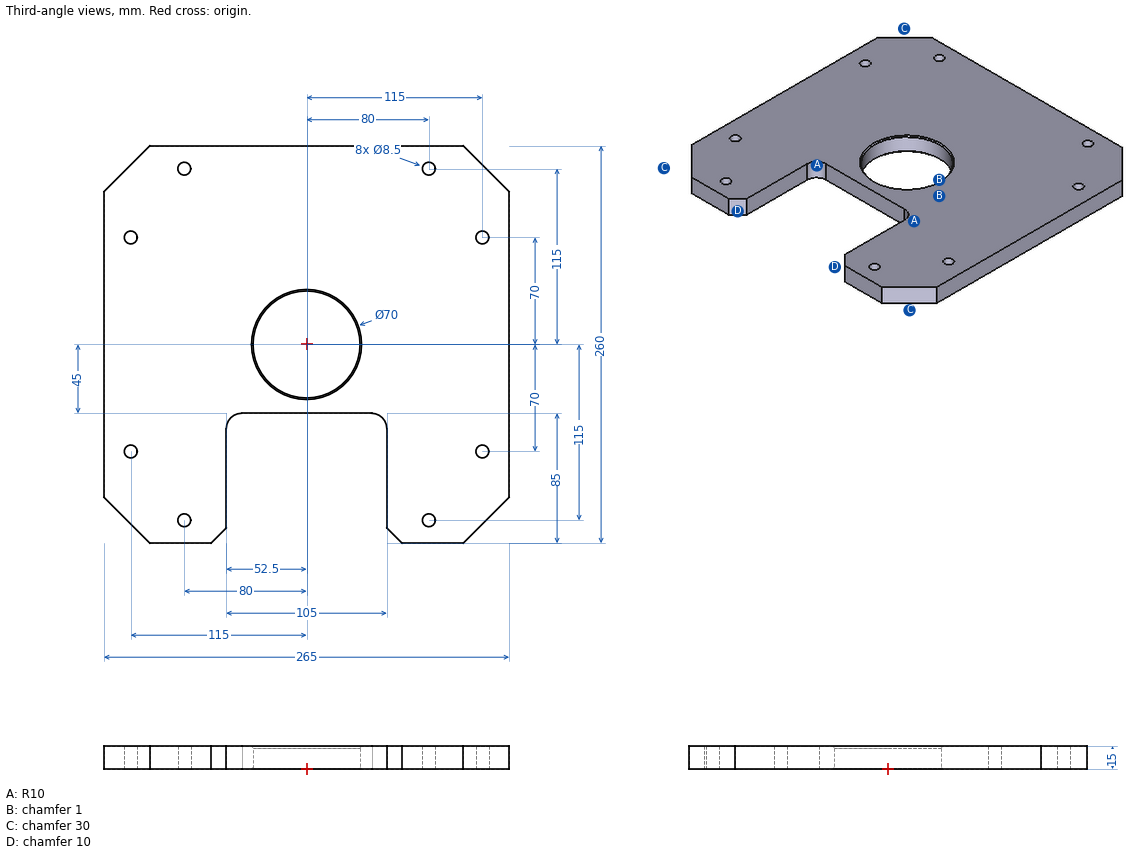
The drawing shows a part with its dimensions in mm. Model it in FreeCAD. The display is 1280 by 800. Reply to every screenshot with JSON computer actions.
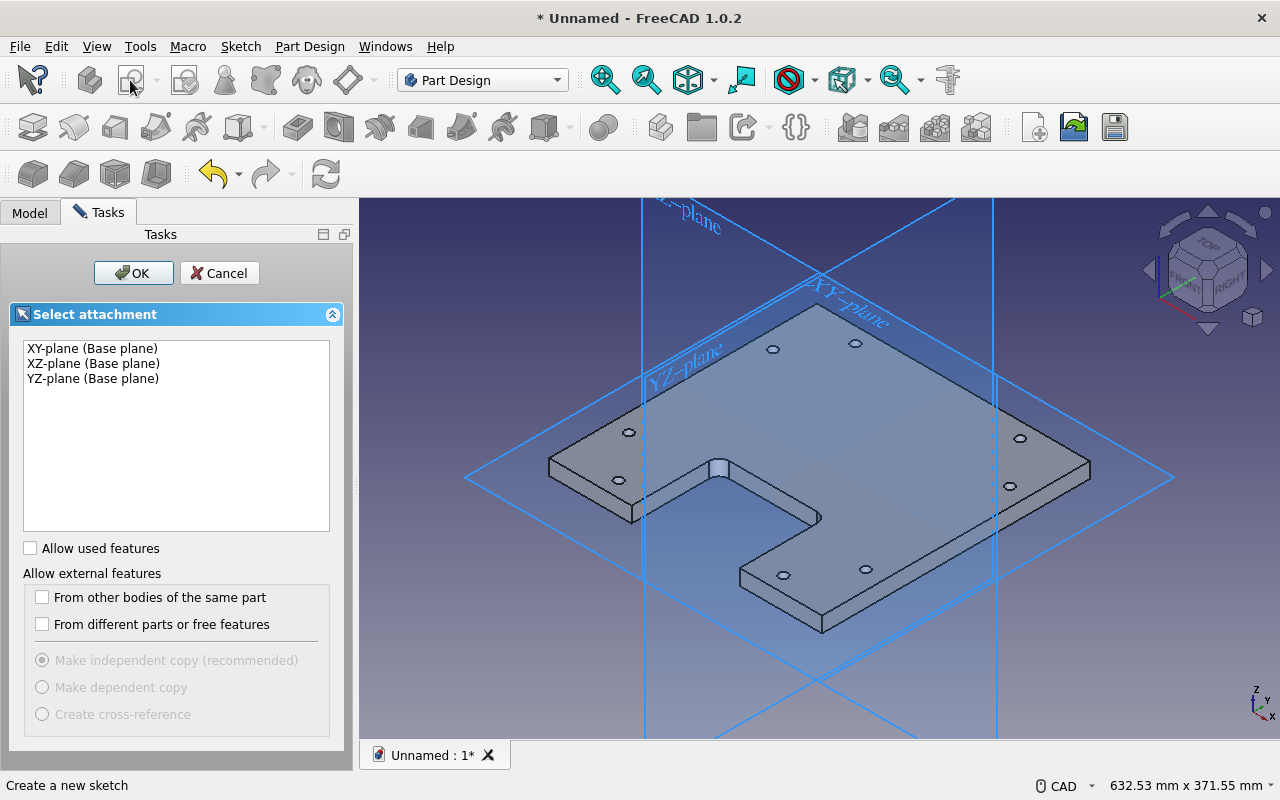
{"action": "left_click", "coordinate": [84, 348]}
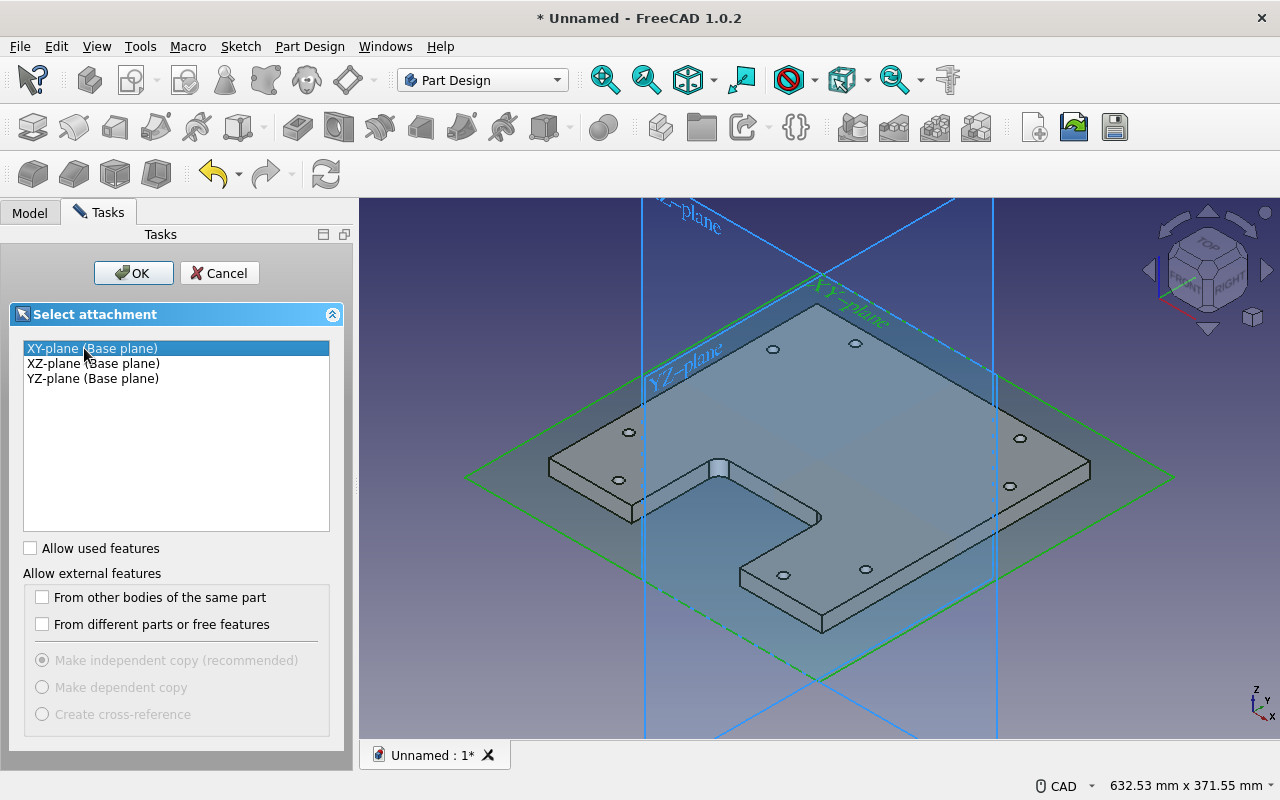
{"action": "left_click", "coordinate": [134, 273]}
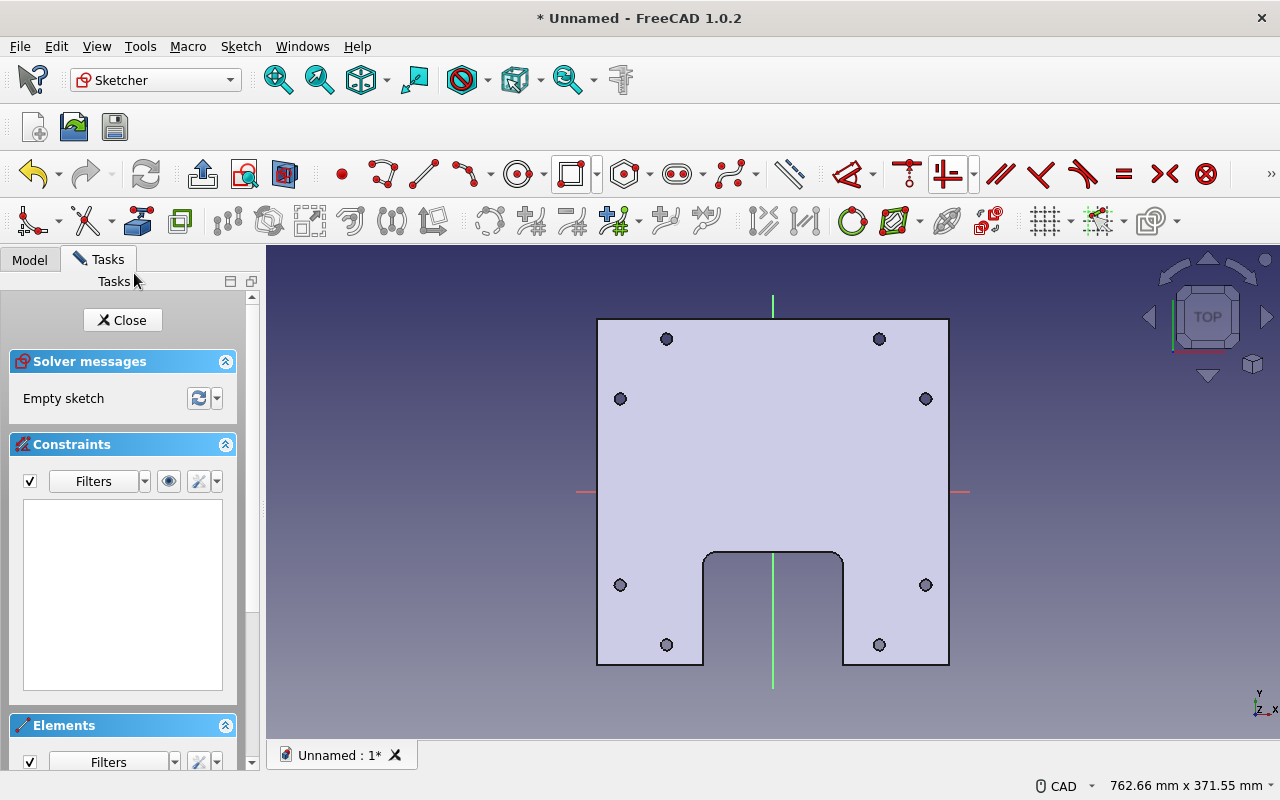
{"action": "key", "text": "q s"}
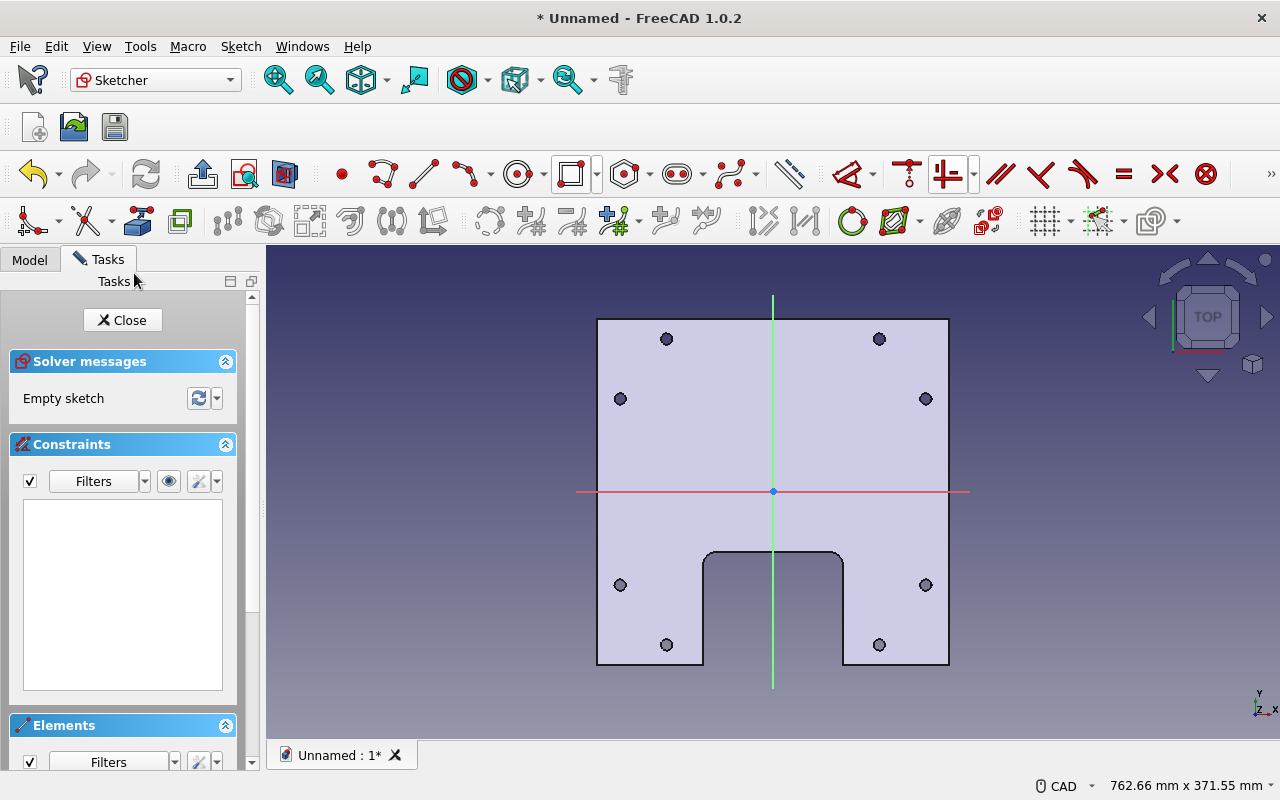
{"action": "scroll", "coordinate": [803, 492], "scroll_direction": "up", "scroll_amount": 6}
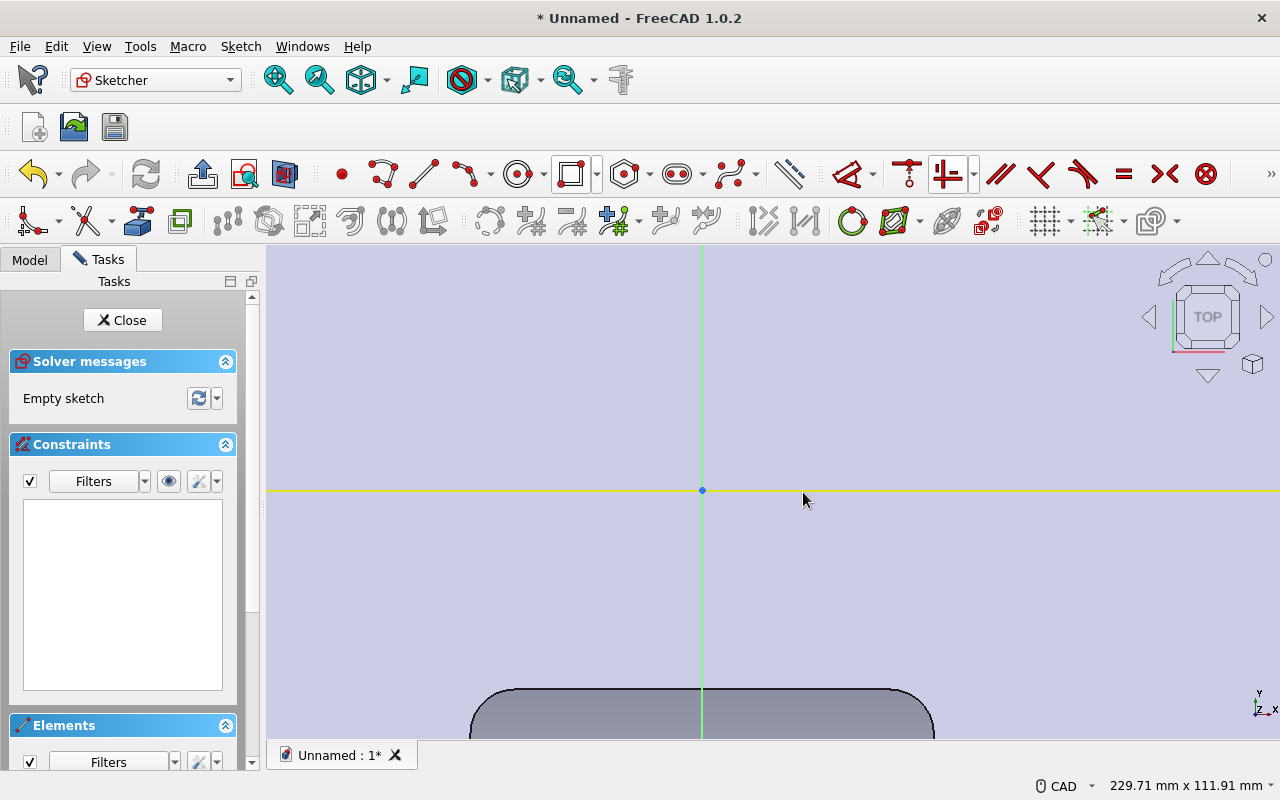
{"action": "left_click", "coordinate": [518, 174]}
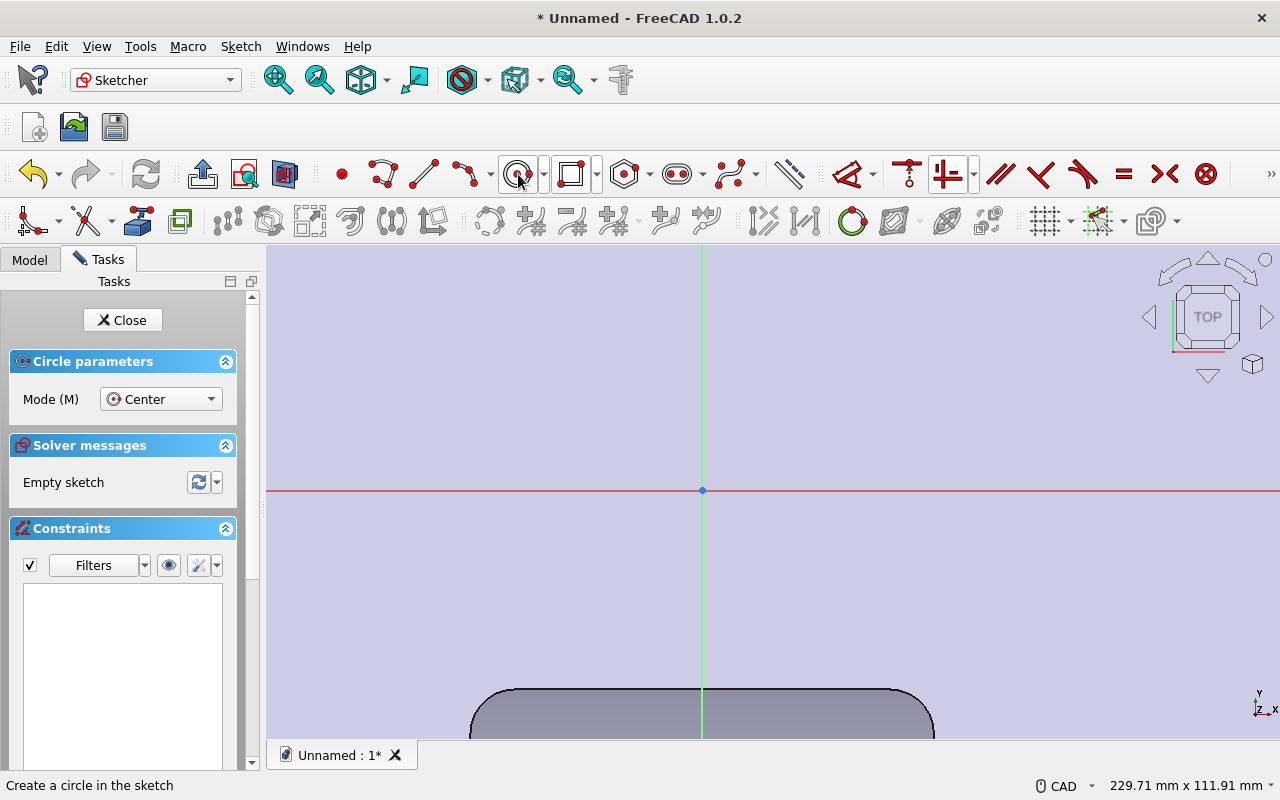
{"action": "left_click", "coordinate": [702, 491]}
{"action": "mouse_move", "coordinate": [811, 382]}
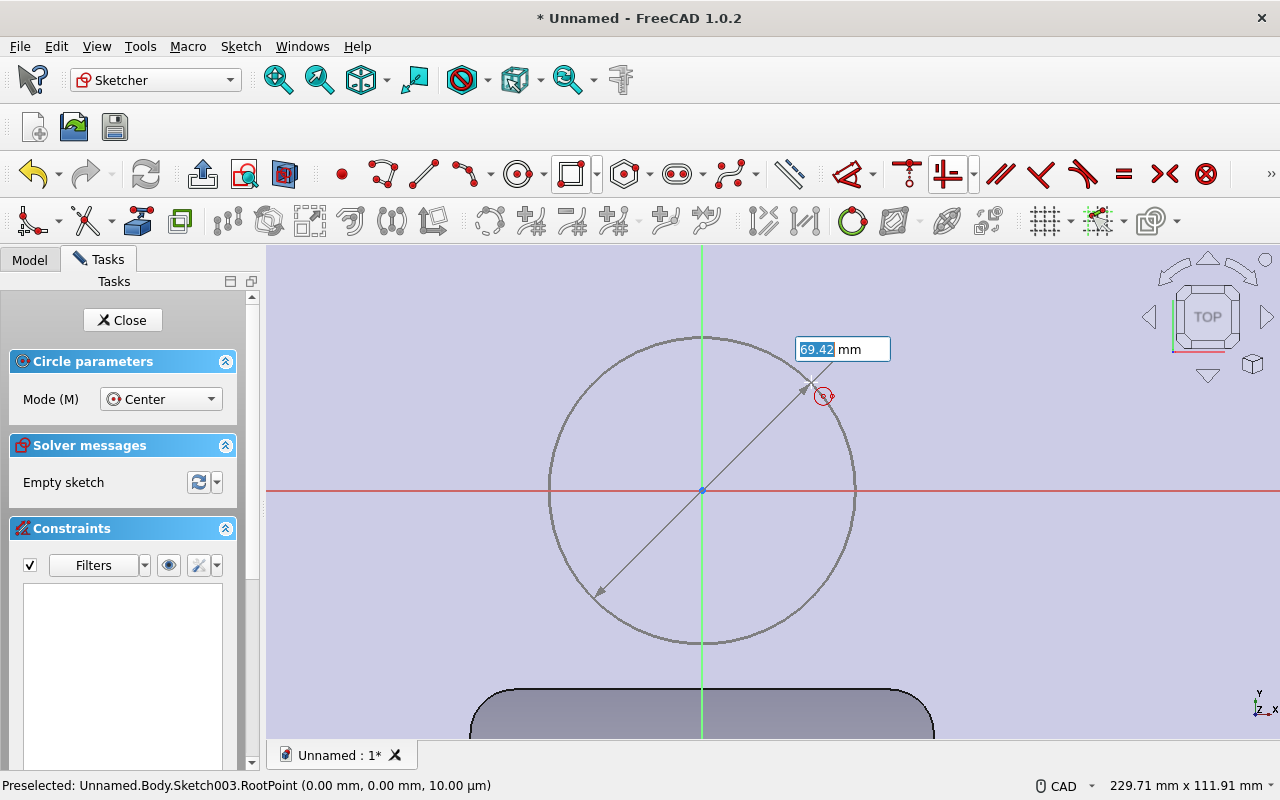
{"action": "type", "text": "70"}
{"action": "key", "text": "Return"}
{"action": "key", "text": "Escape"}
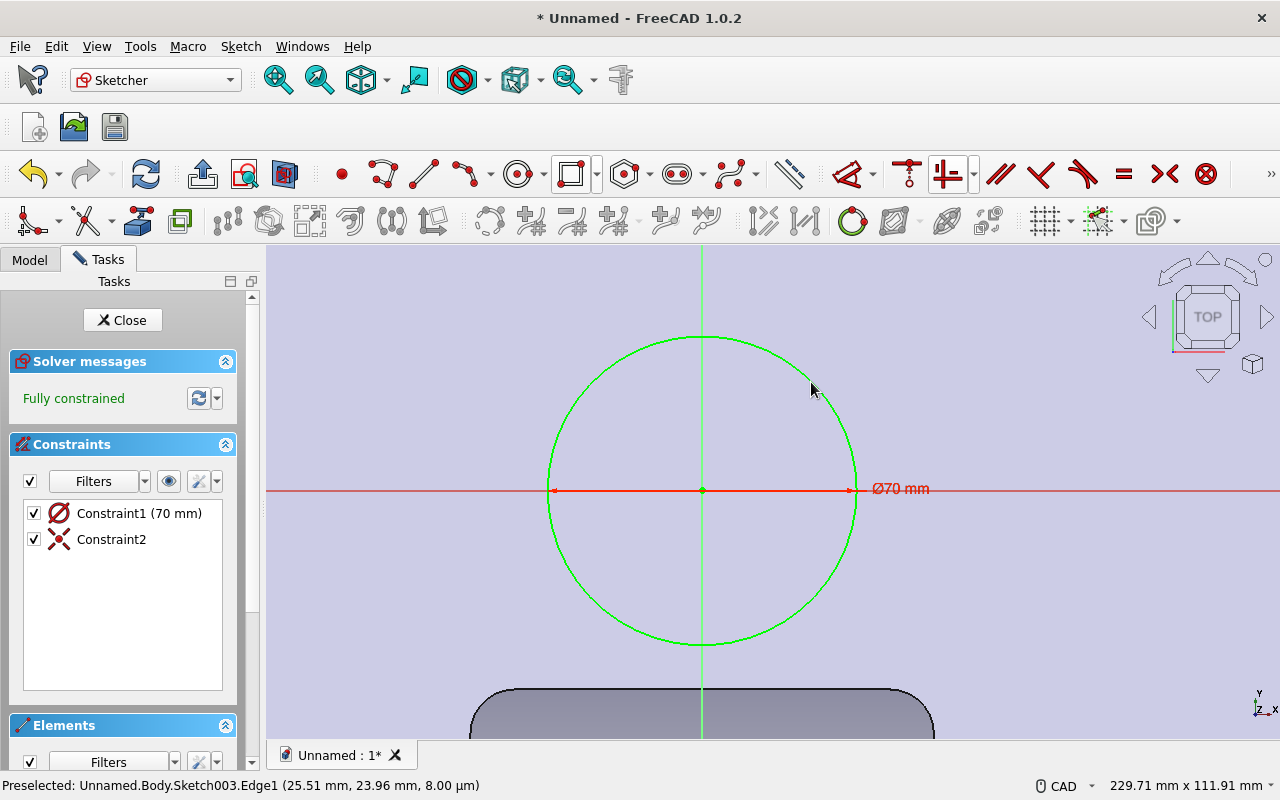
{"action": "left_click", "coordinate": [123, 320]}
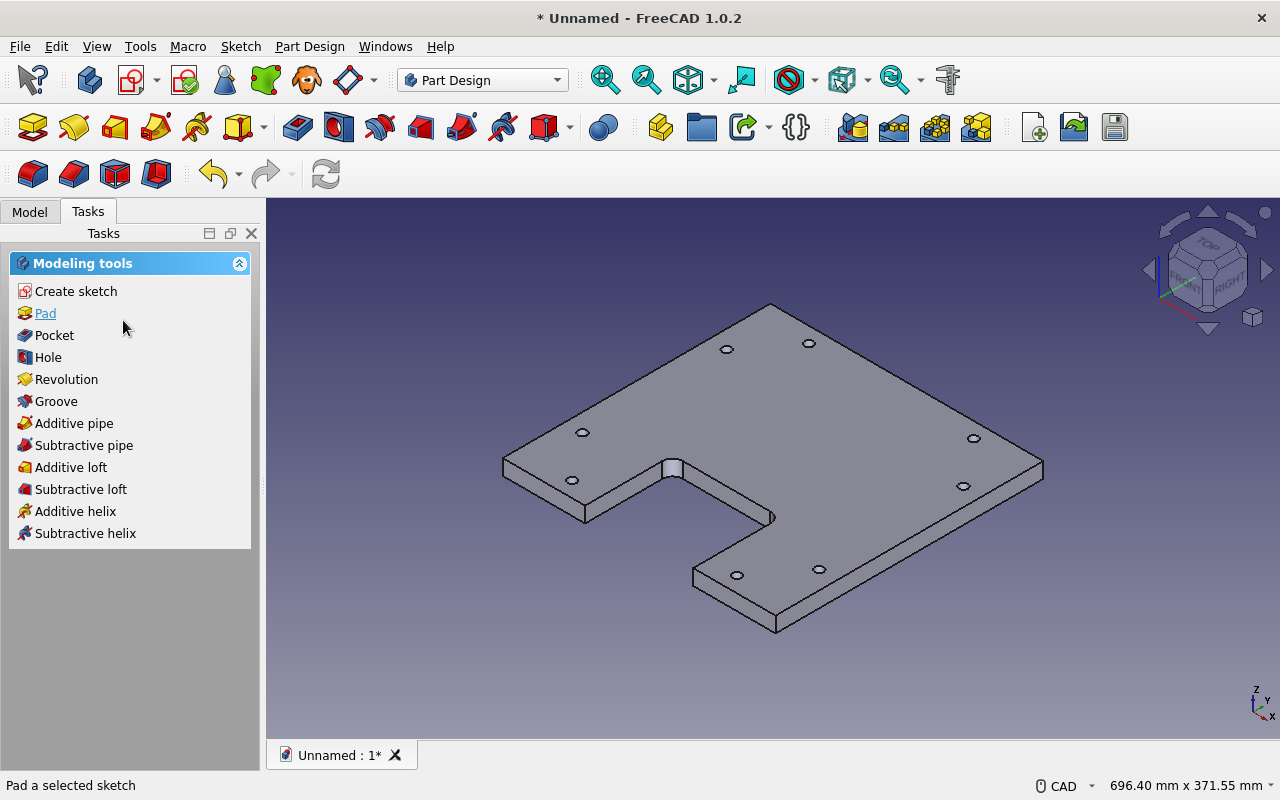
{"action": "left_click", "coordinate": [298, 128]}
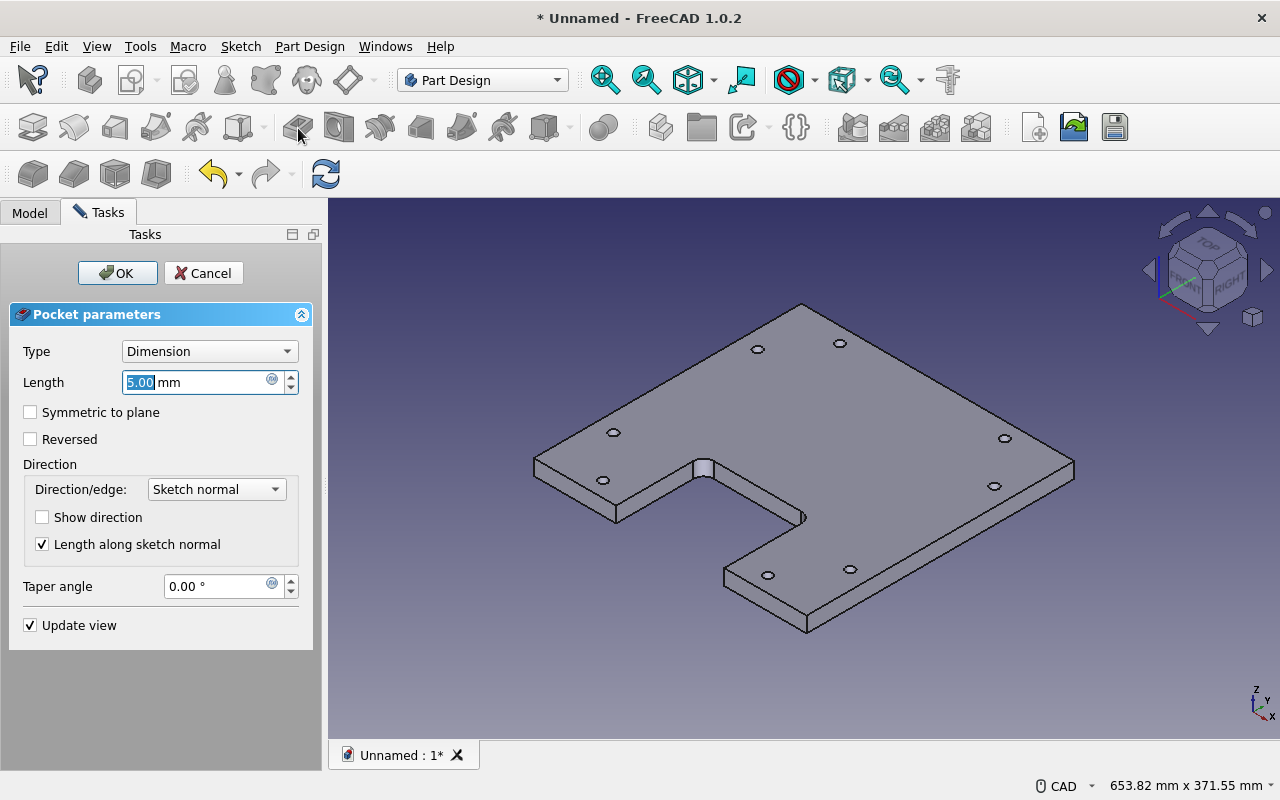
{"action": "left_click", "coordinate": [210, 352]}